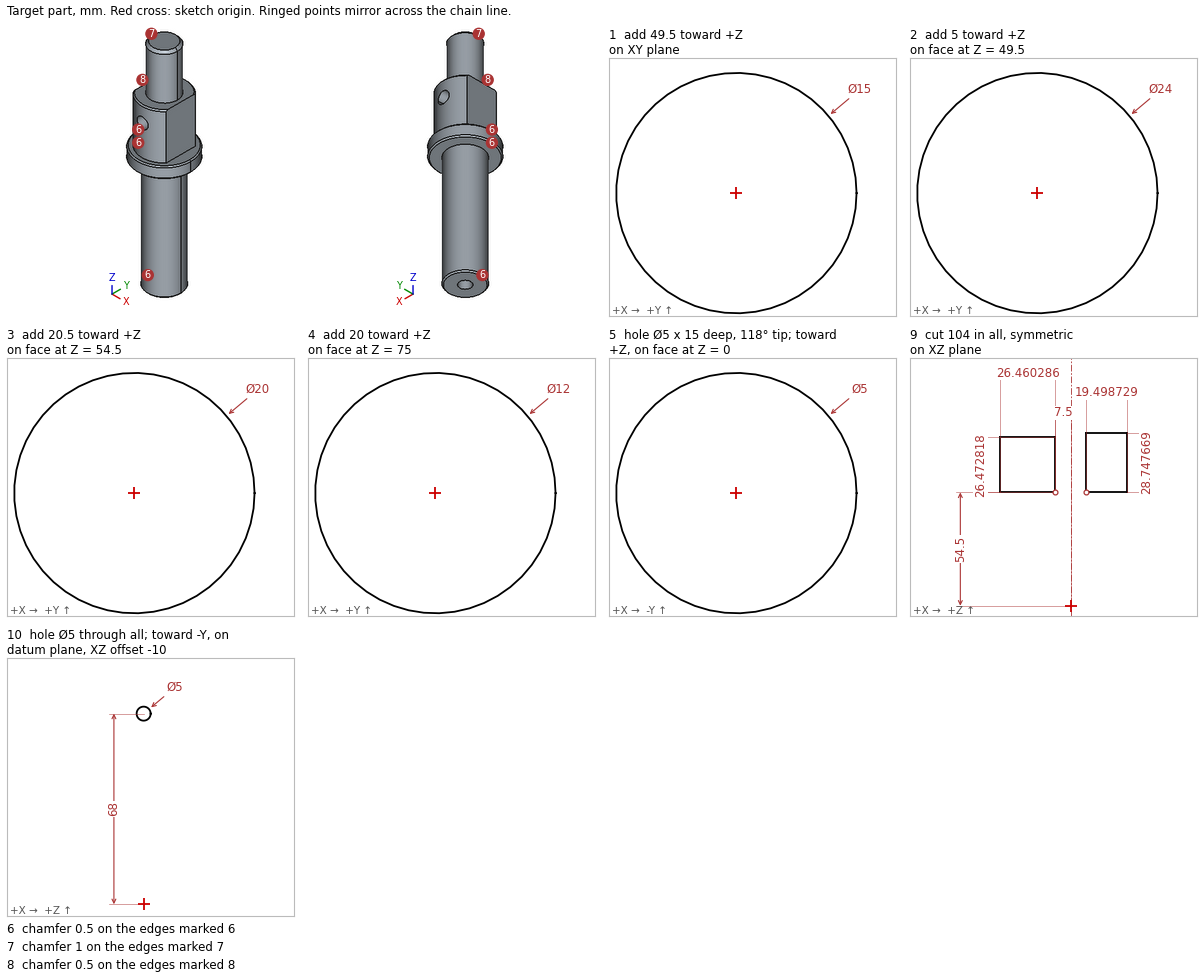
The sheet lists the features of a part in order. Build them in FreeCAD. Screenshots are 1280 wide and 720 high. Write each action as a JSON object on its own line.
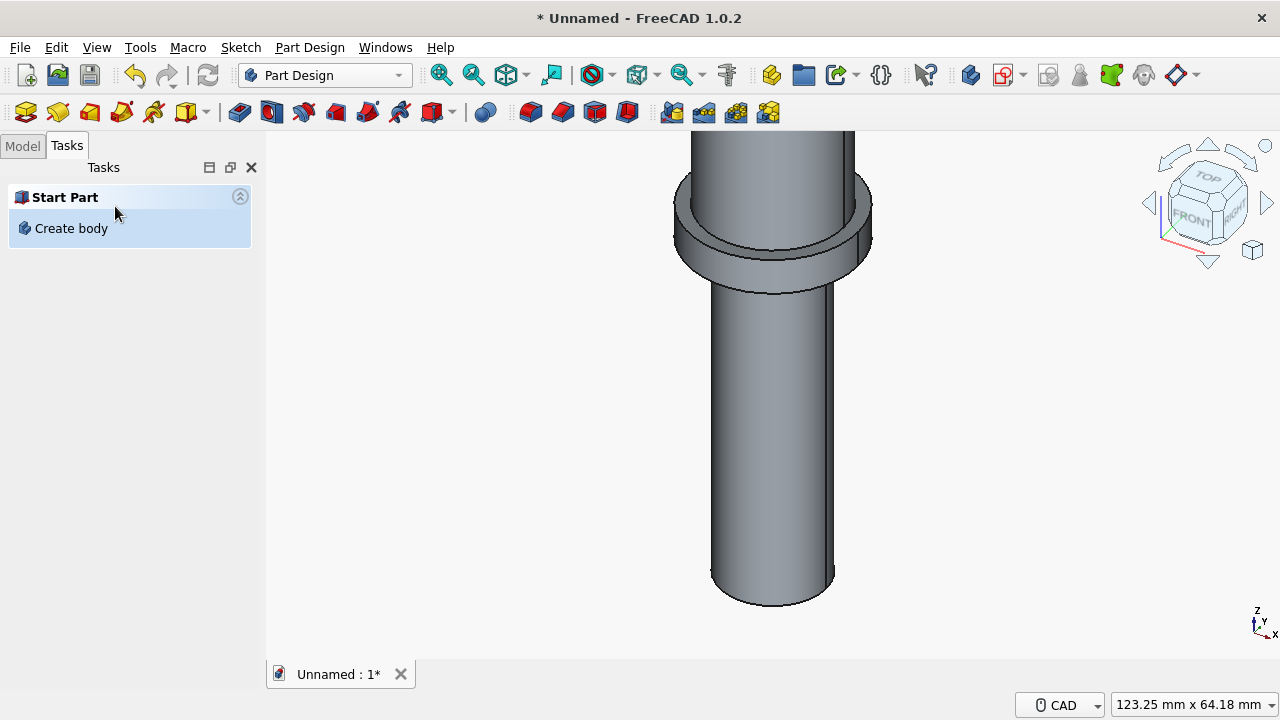
{"action": "key", "text": "v f"}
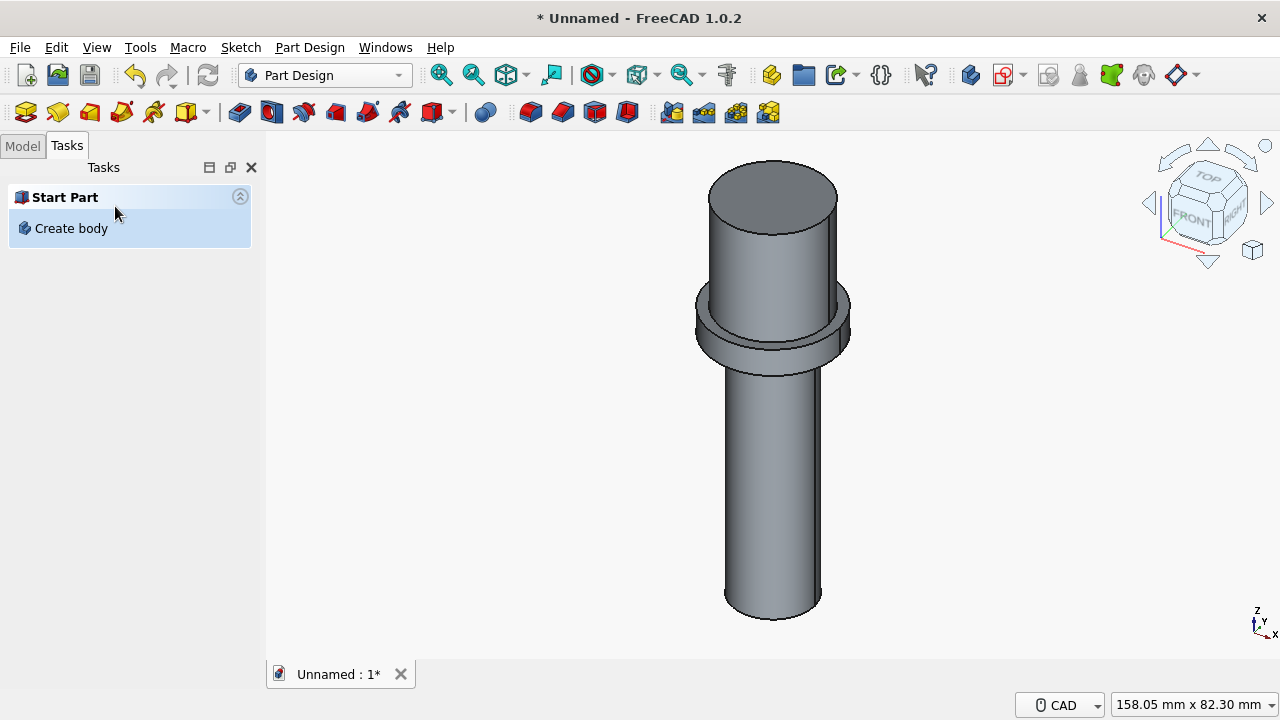
{"action": "left_click", "coordinate": [773, 197]}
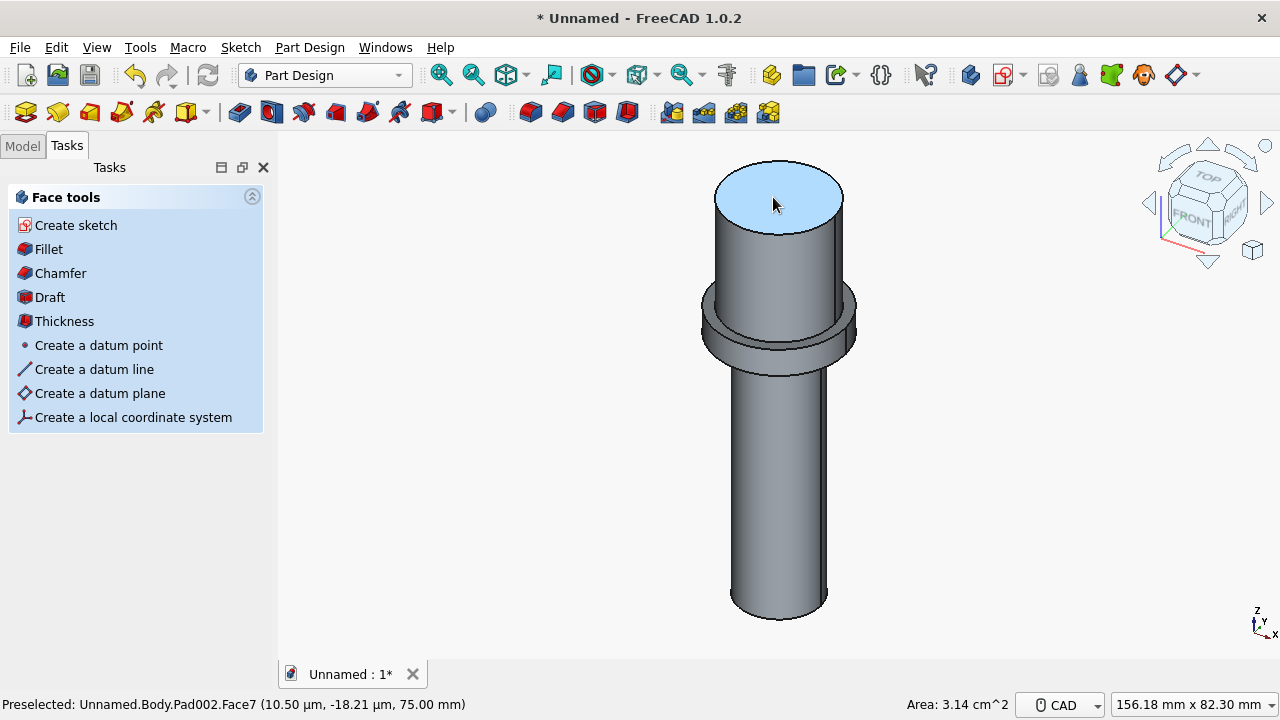
{"action": "left_click", "coordinate": [1004, 76]}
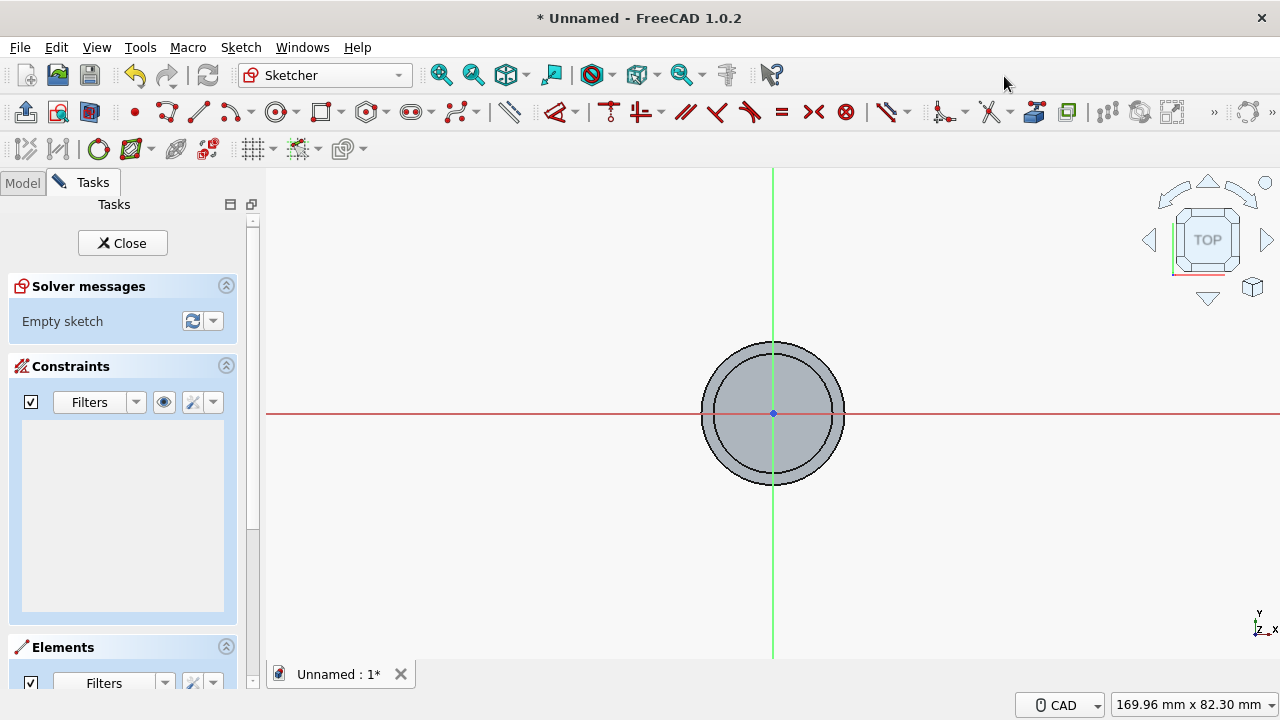
{"action": "scroll", "coordinate": [795, 414], "scroll_direction": "up", "scroll_amount": 7}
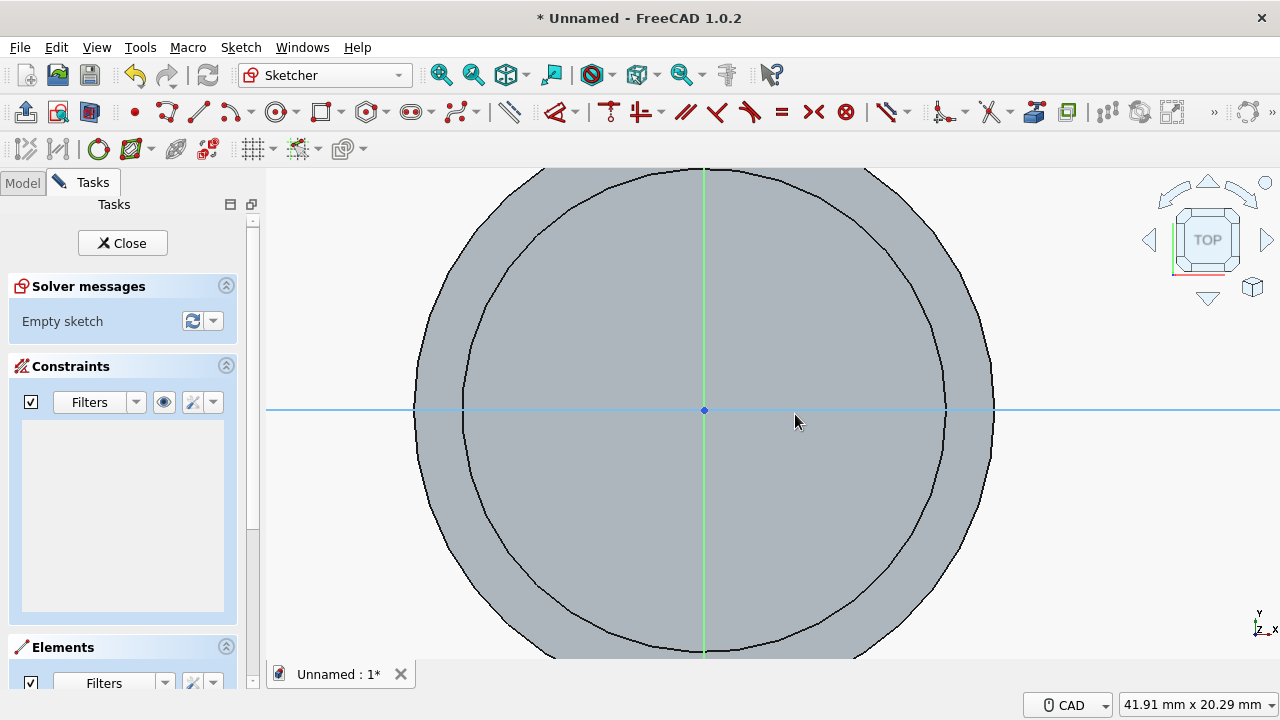
{"action": "key", "text": "g c"}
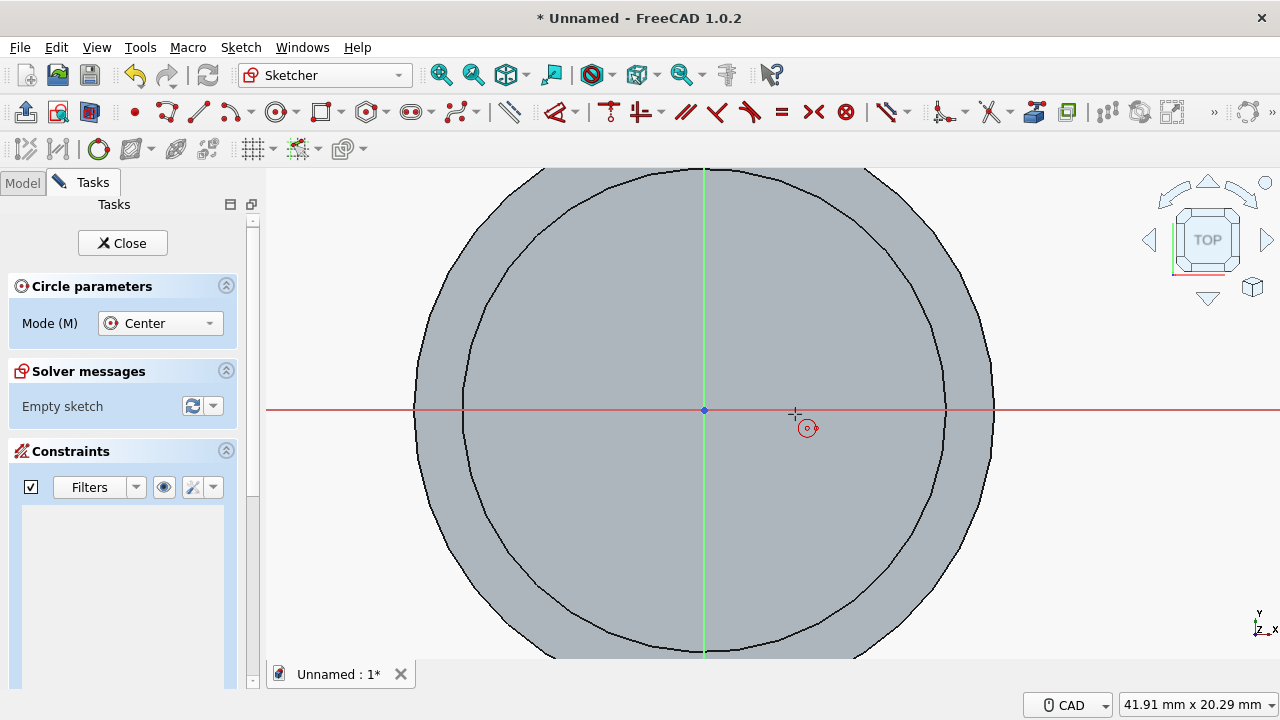
{"action": "left_click", "coordinate": [704, 410]}
{"action": "mouse_move", "coordinate": [807, 308]}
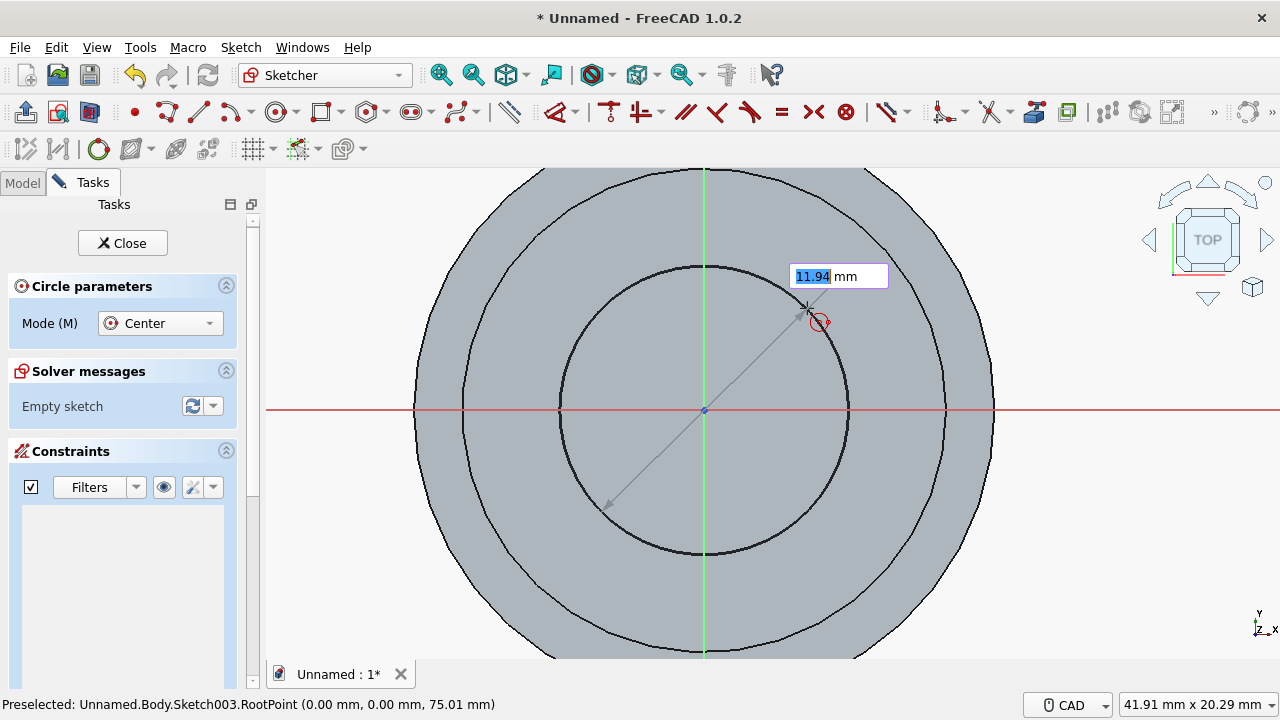
{"action": "type", "text": "12"}
{"action": "key", "text": "Return"}
{"action": "key", "text": "Escape"}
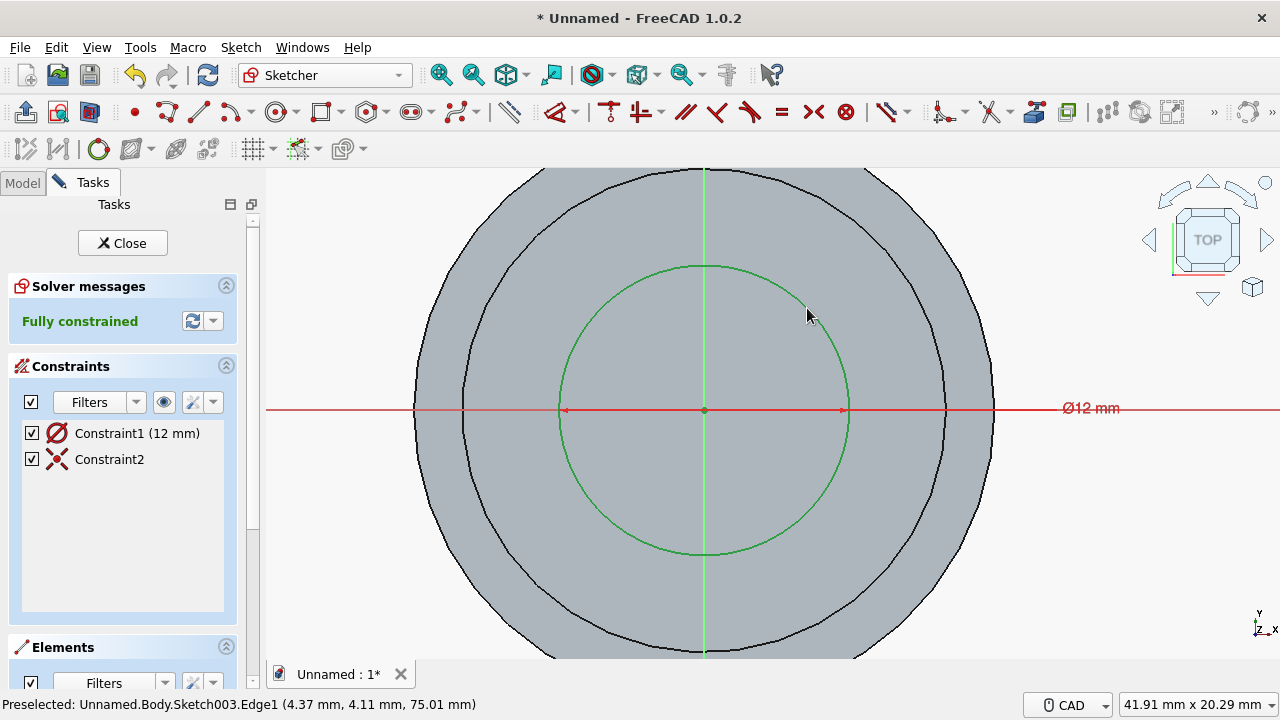
{"action": "left_click", "coordinate": [123, 243]}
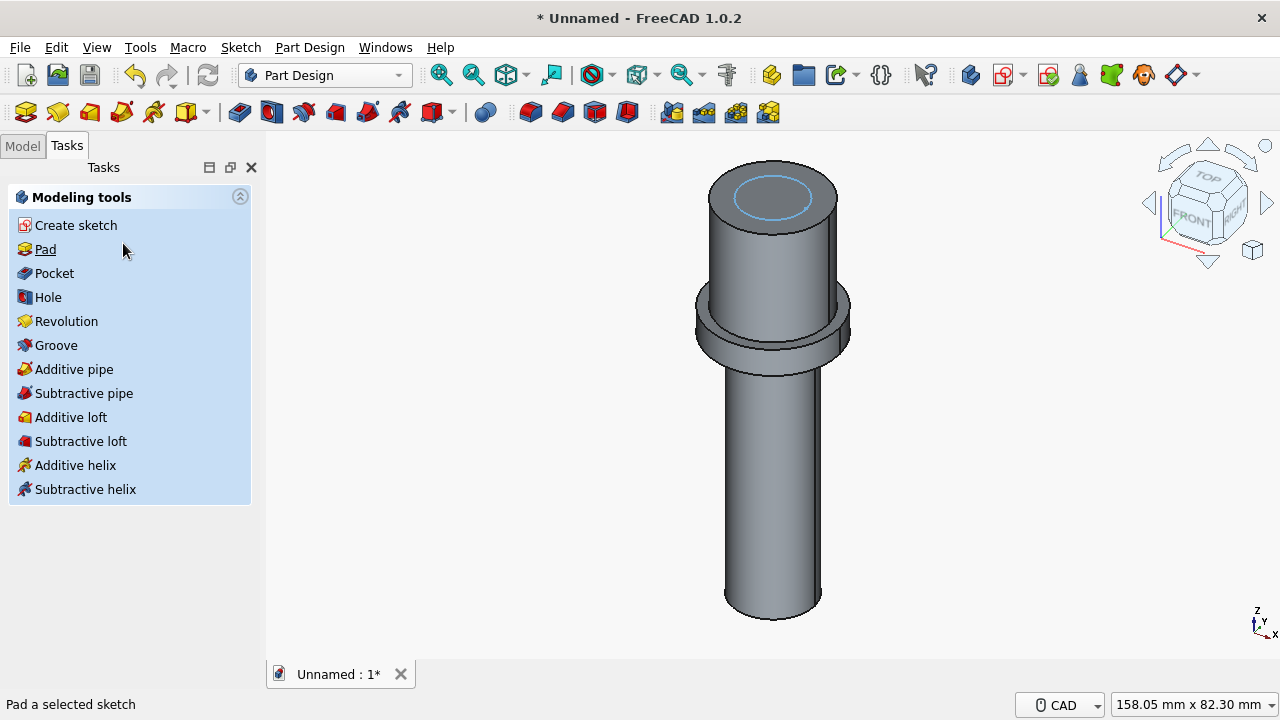
{"action": "left_click", "coordinate": [26, 112]}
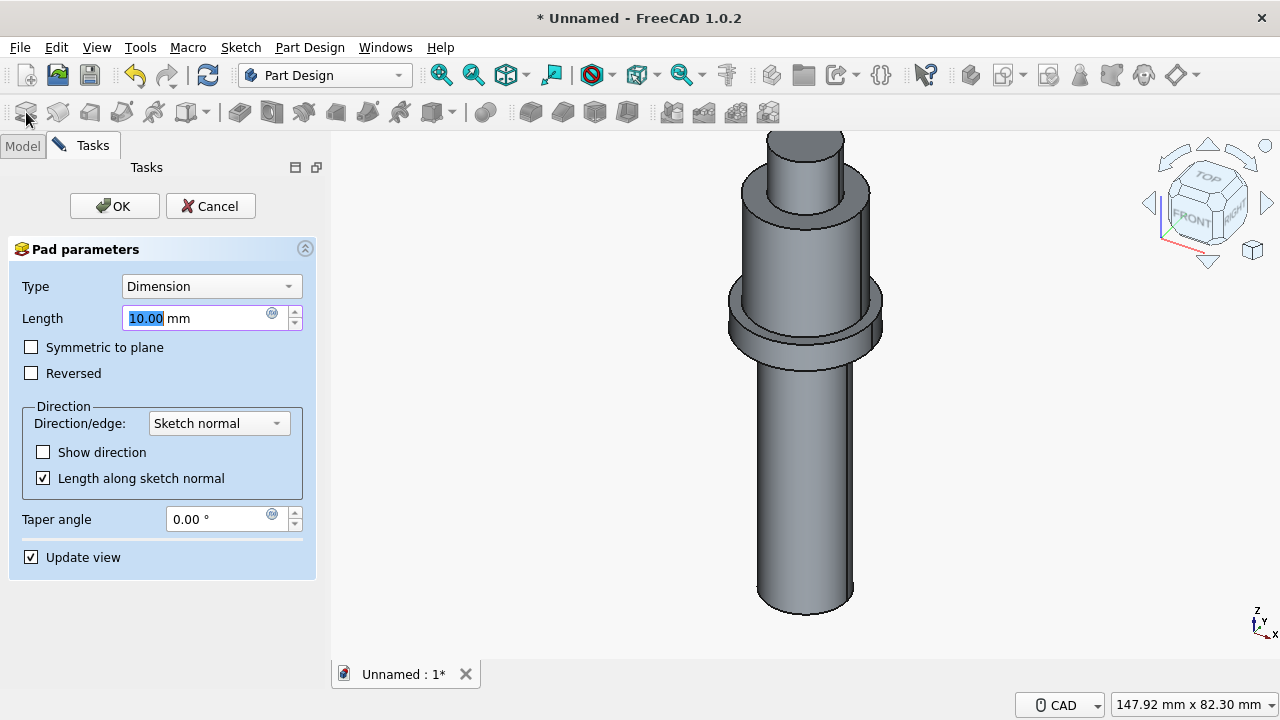
{"action": "type", "text": "20"}
{"action": "key", "text": "Tab"}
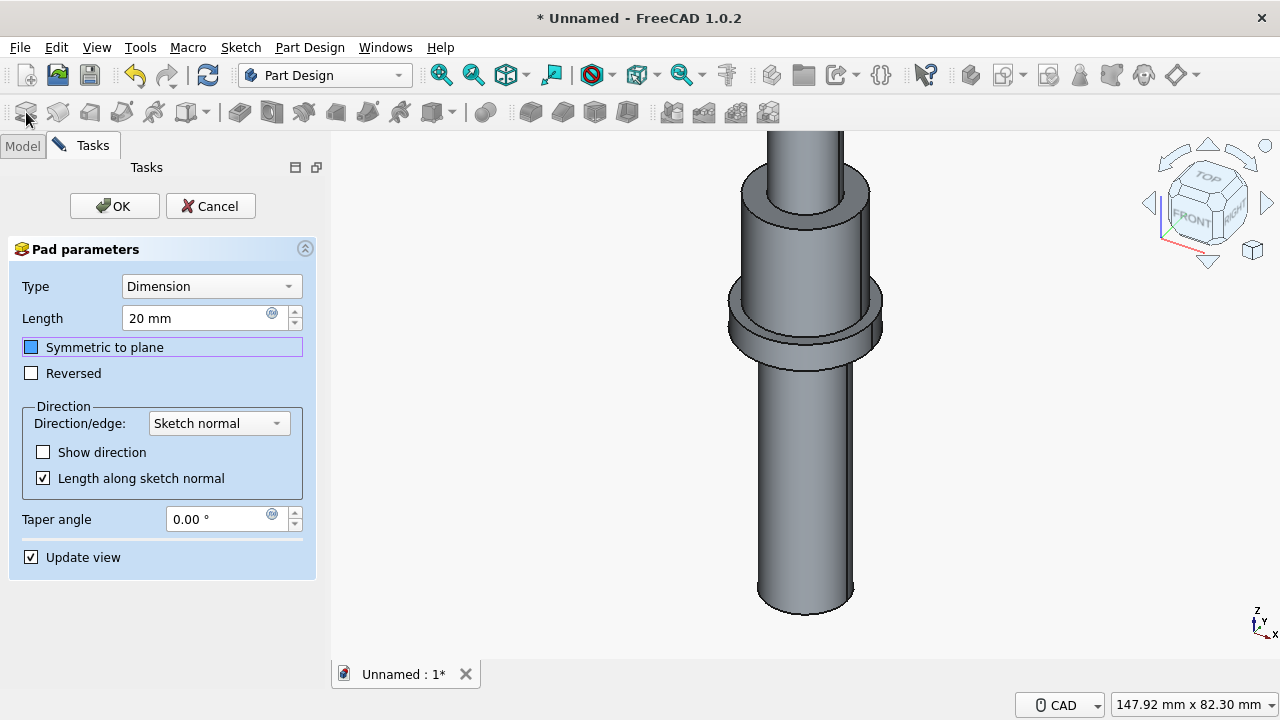
{"action": "left_click", "coordinate": [115, 206]}